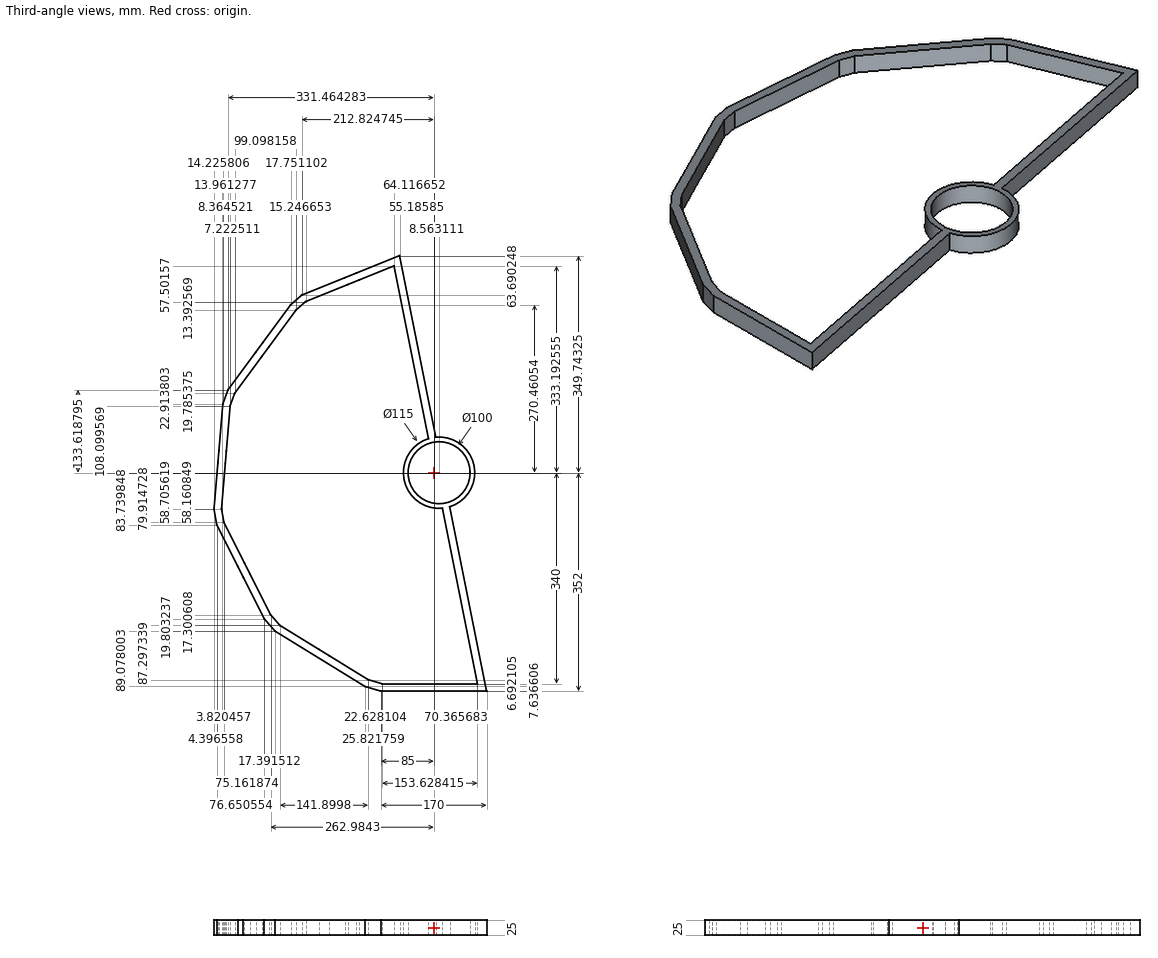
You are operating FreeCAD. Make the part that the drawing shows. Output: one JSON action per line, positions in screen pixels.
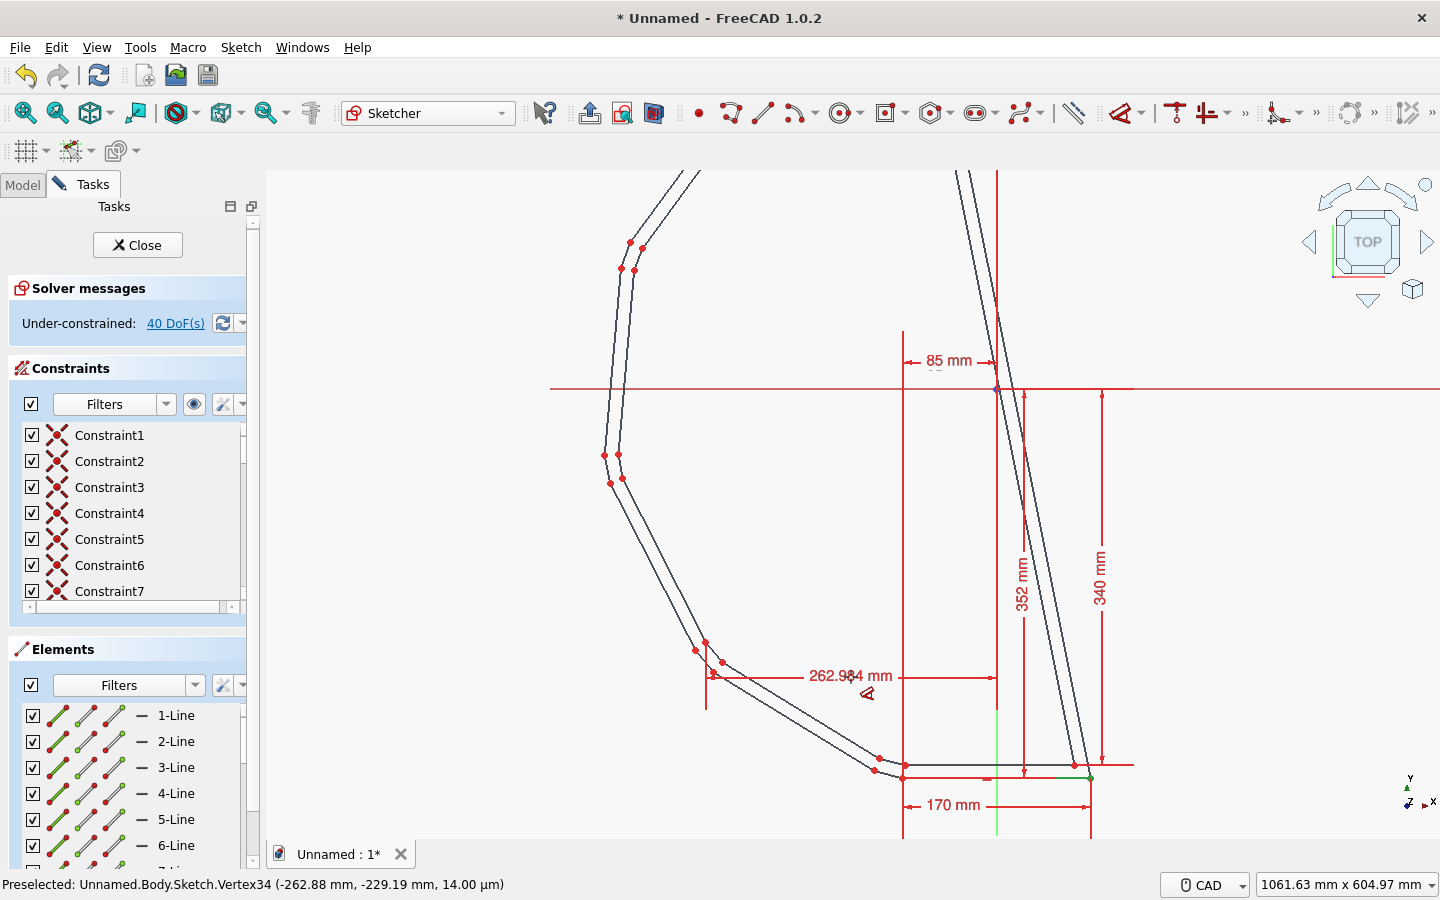
{"action": "scroll", "coordinate": [627, 253], "scroll_direction": "up", "scroll_amount": 8}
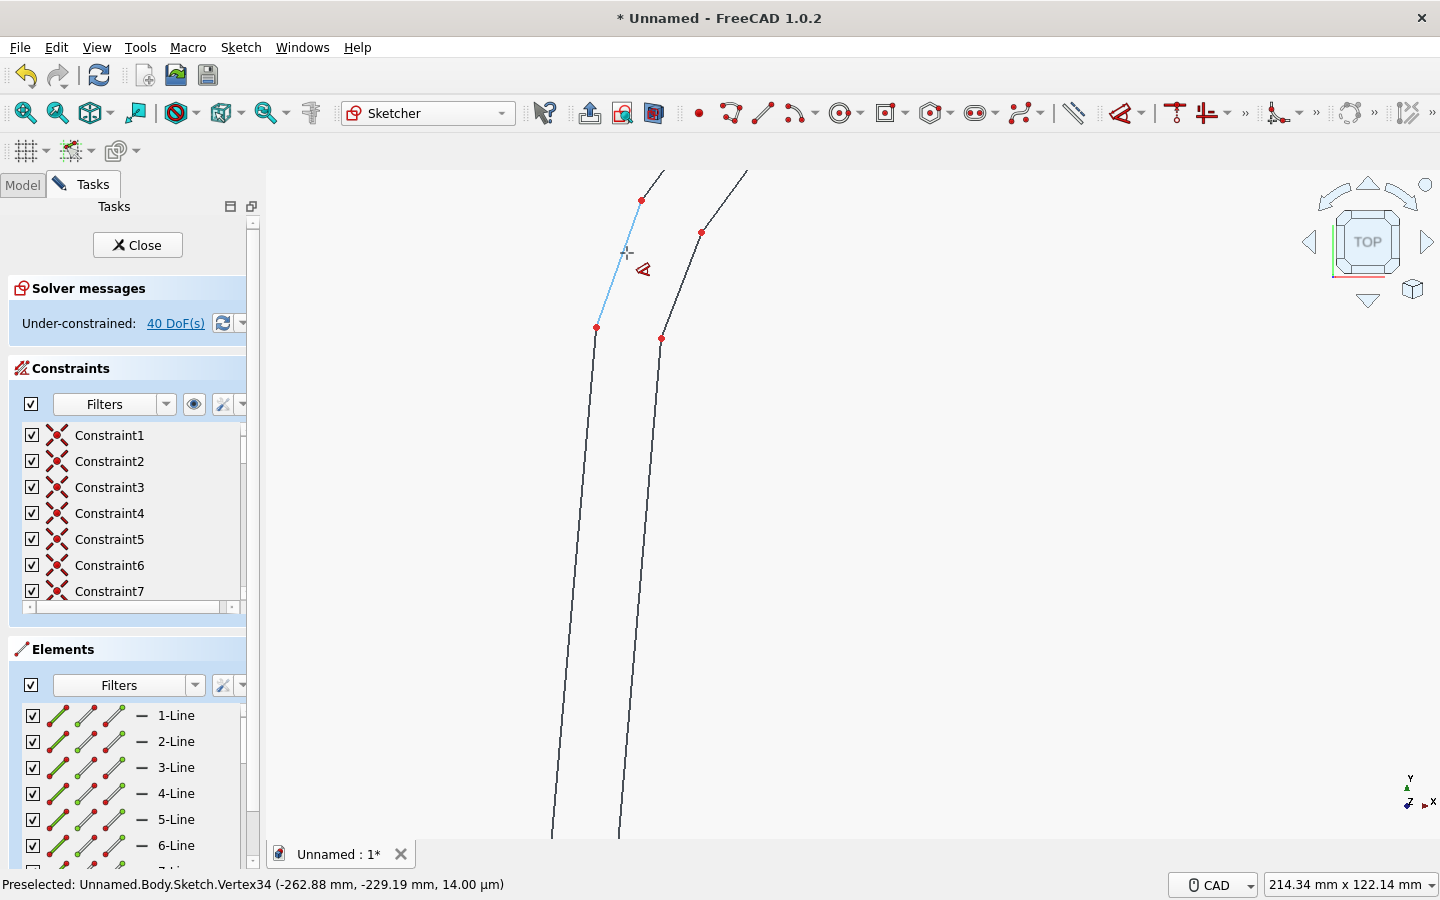
{"action": "left_click", "coordinate": [623, 251]}
{"action": "left_click", "coordinate": [619, 361]}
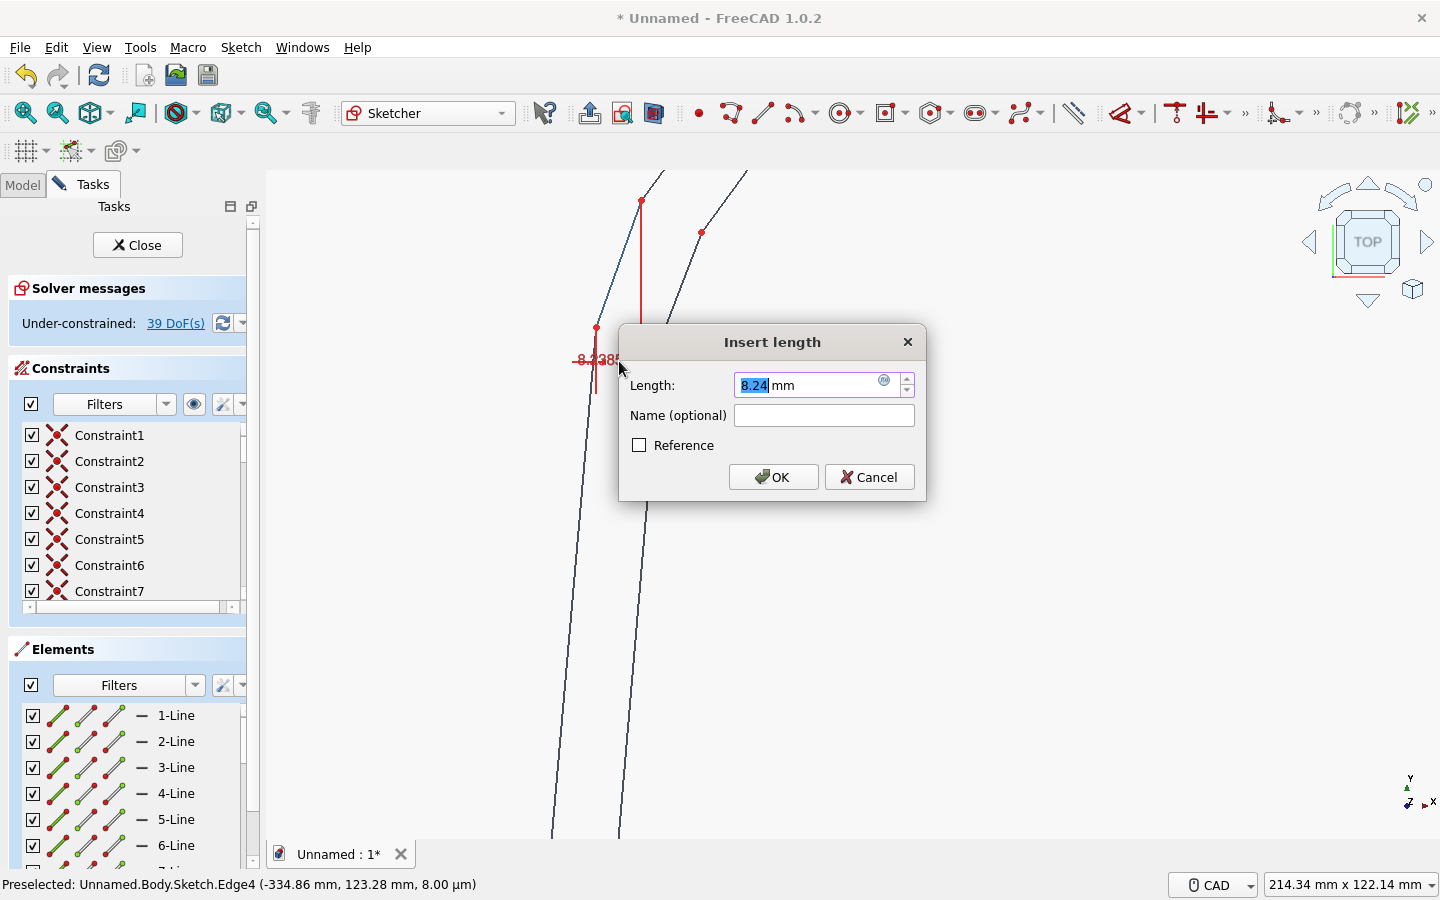
{"action": "type", "text": "8.364521"}
{"action": "key", "text": "Return"}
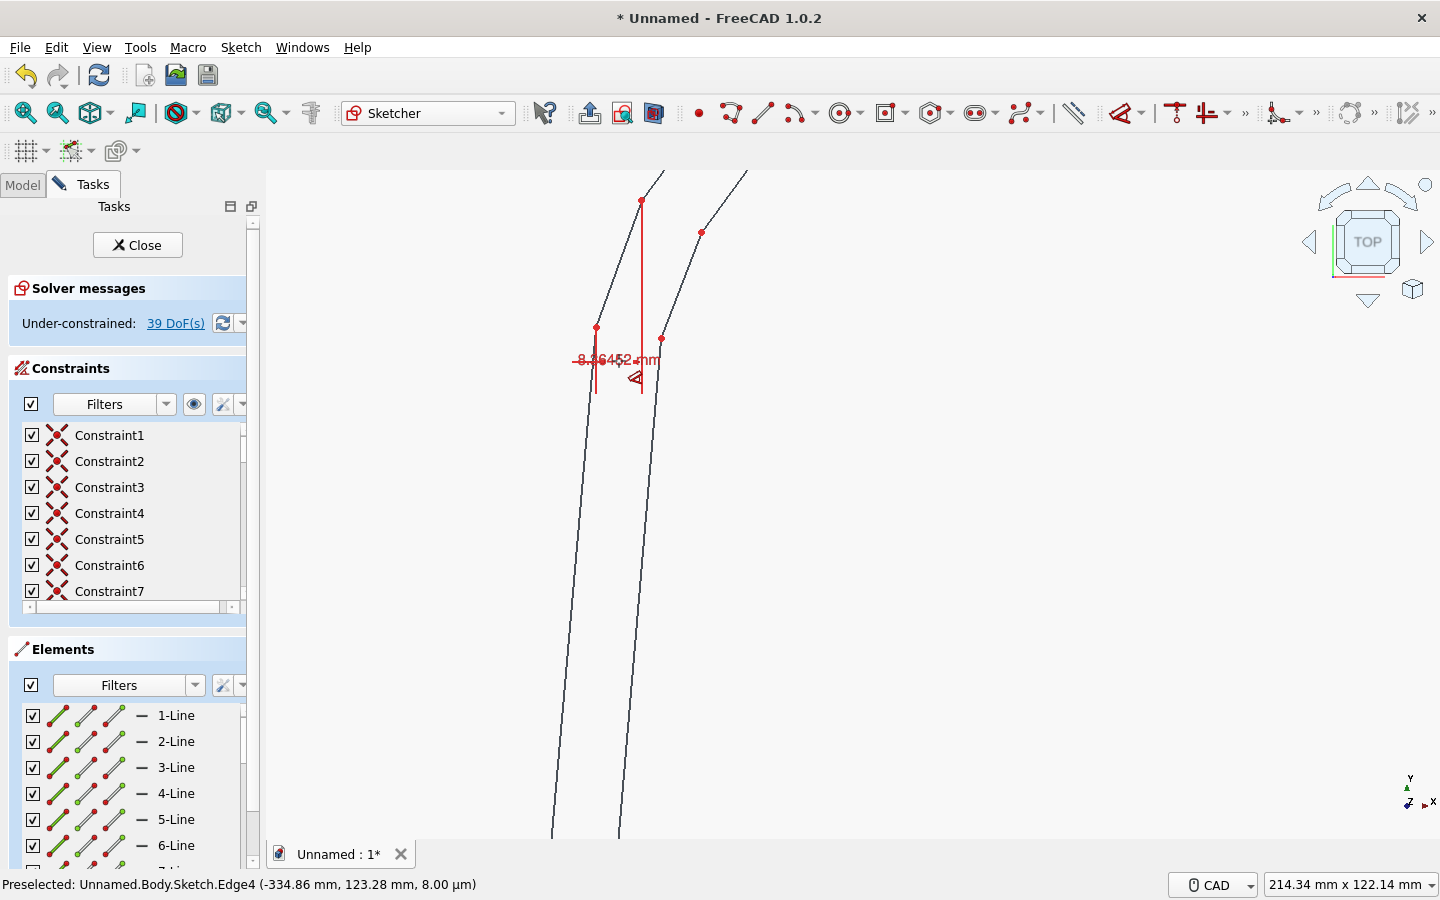
{"action": "scroll", "coordinate": [668, 451], "scroll_direction": "down", "scroll_amount": 11}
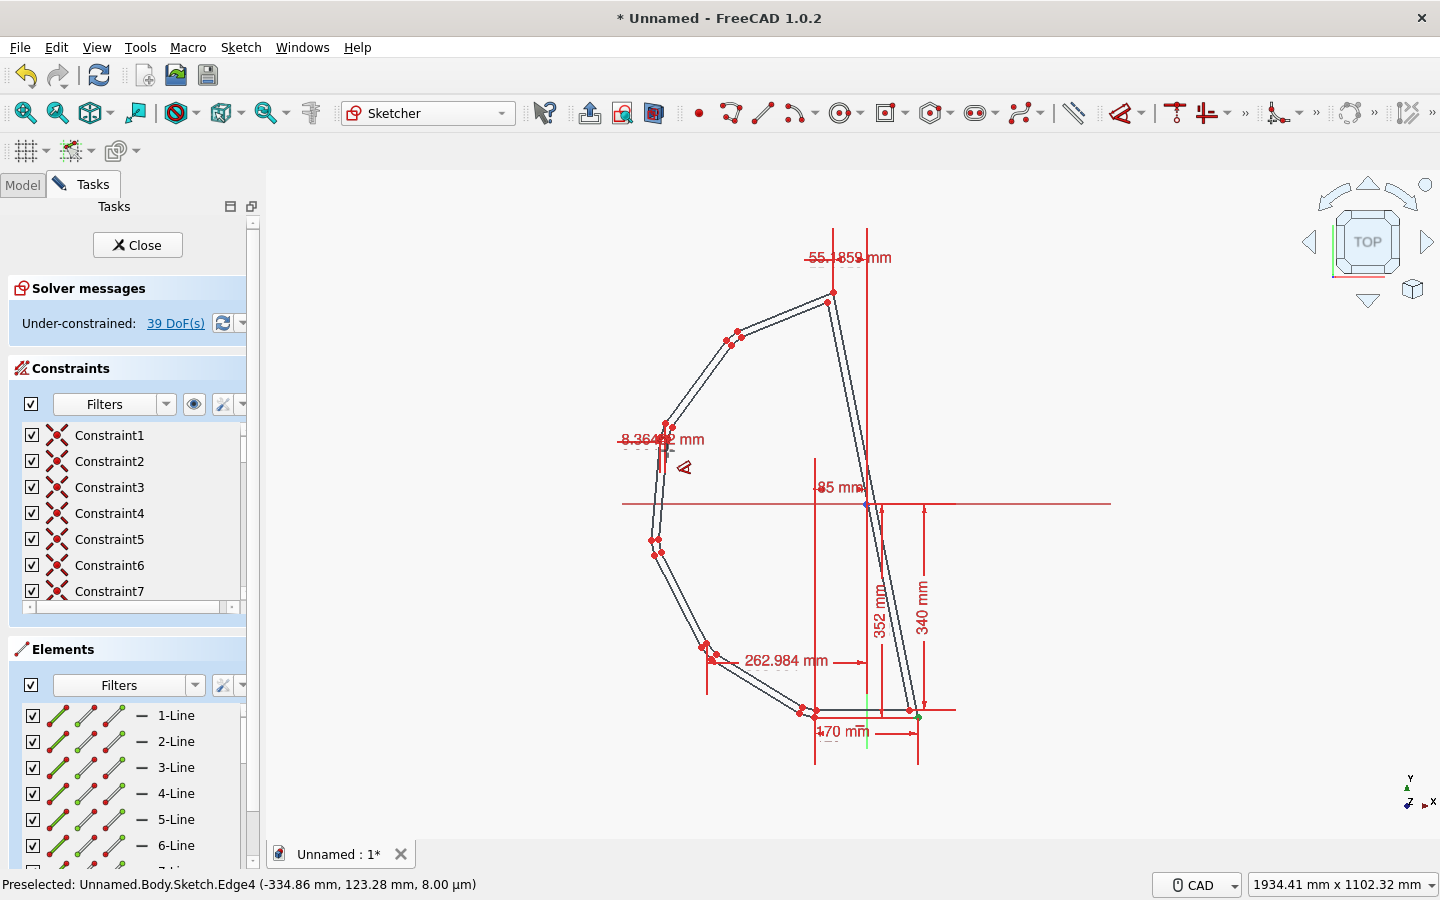
{"action": "scroll", "coordinate": [652, 545], "scroll_direction": "up", "scroll_amount": 14}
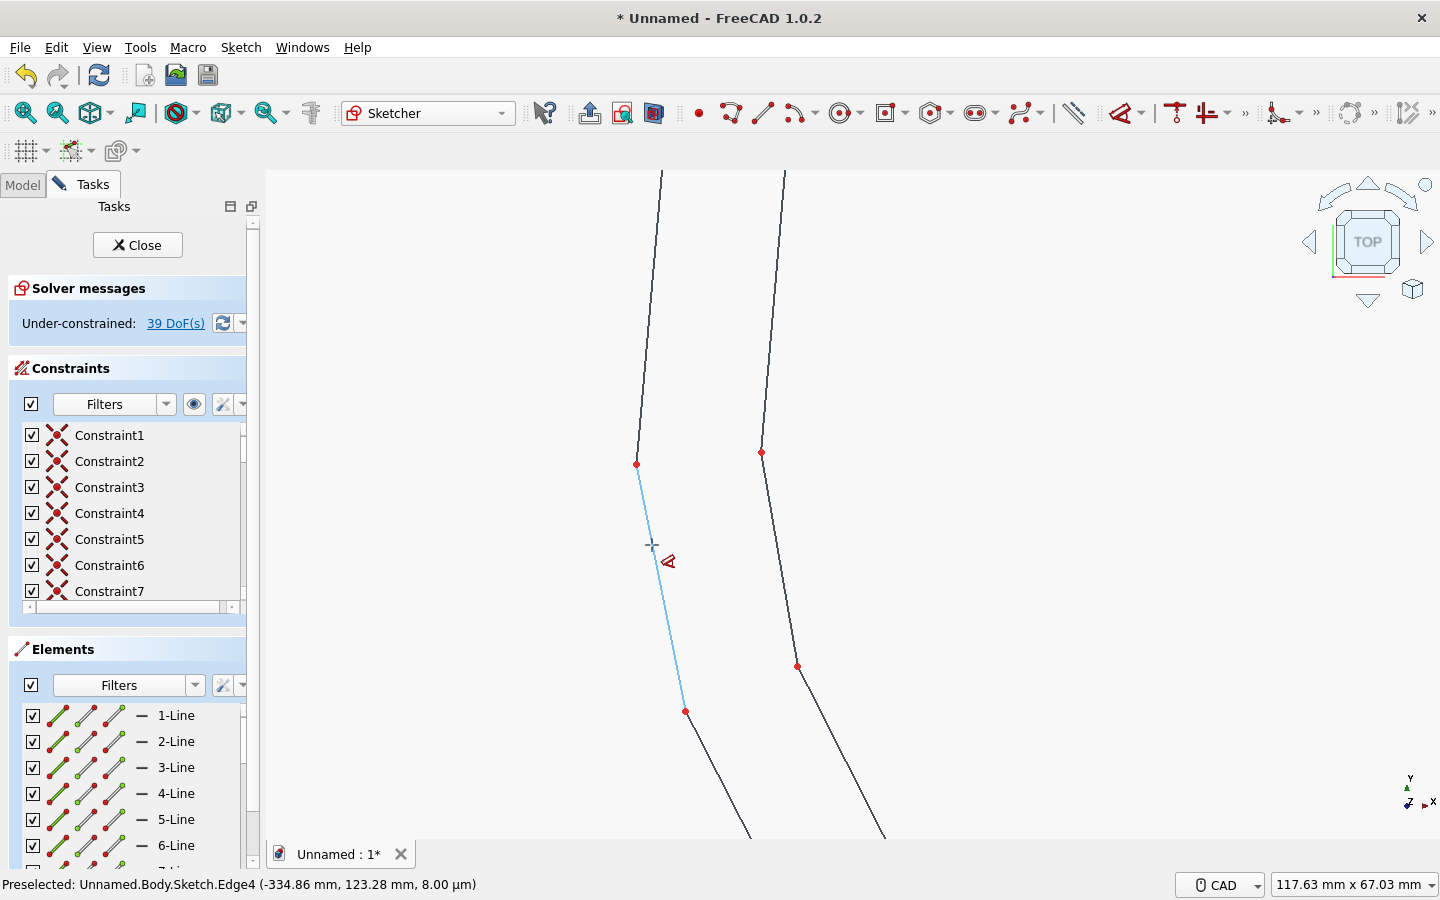
{"action": "left_click", "coordinate": [651, 539]}
{"action": "left_click", "coordinate": [661, 745]}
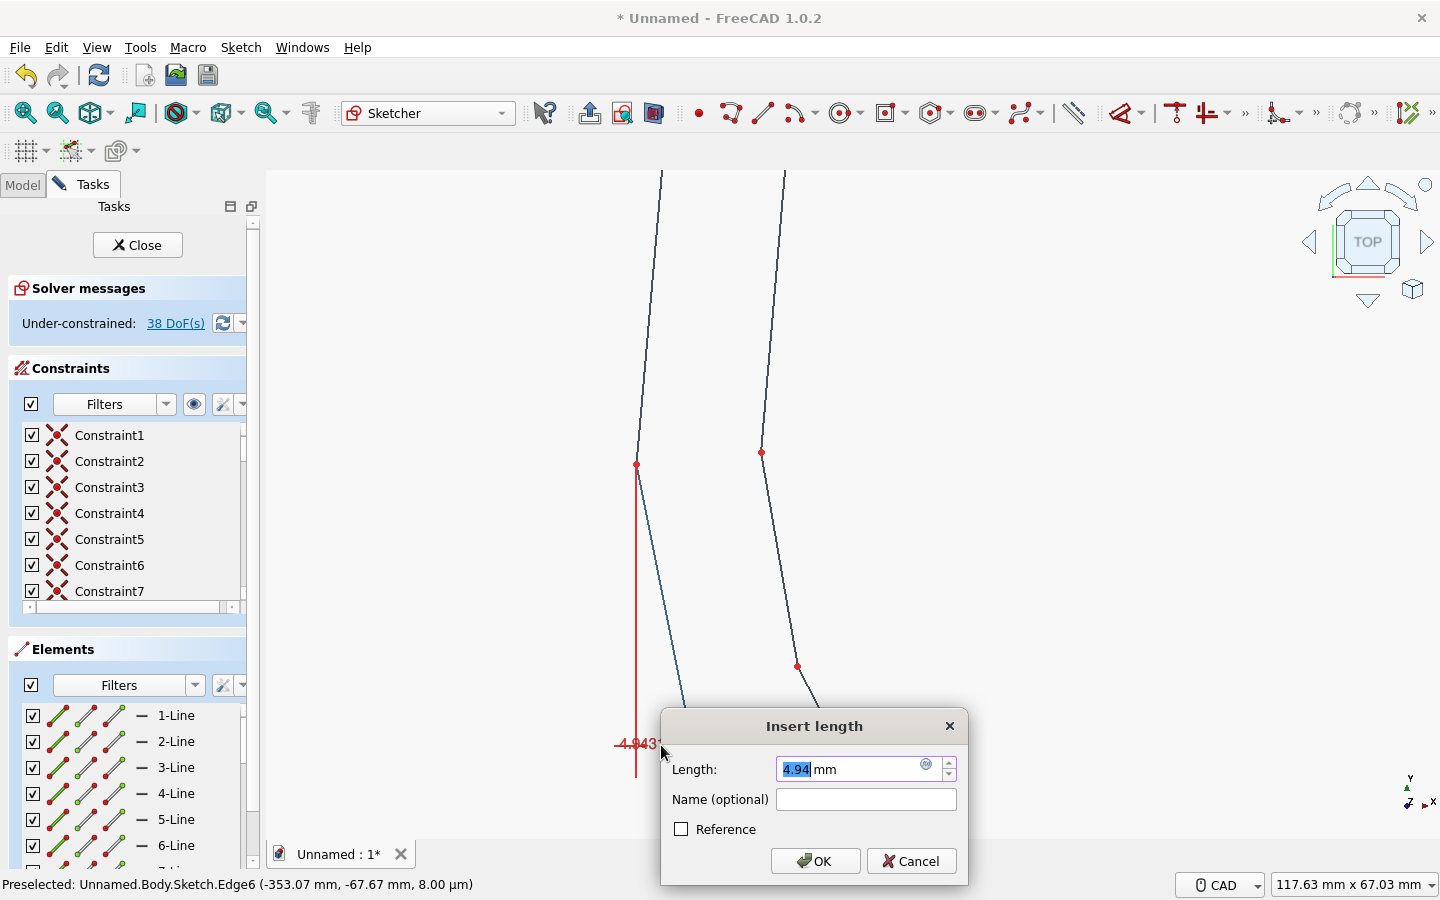
{"action": "type", "text": "4.396558"}
{"action": "key", "text": "Return"}